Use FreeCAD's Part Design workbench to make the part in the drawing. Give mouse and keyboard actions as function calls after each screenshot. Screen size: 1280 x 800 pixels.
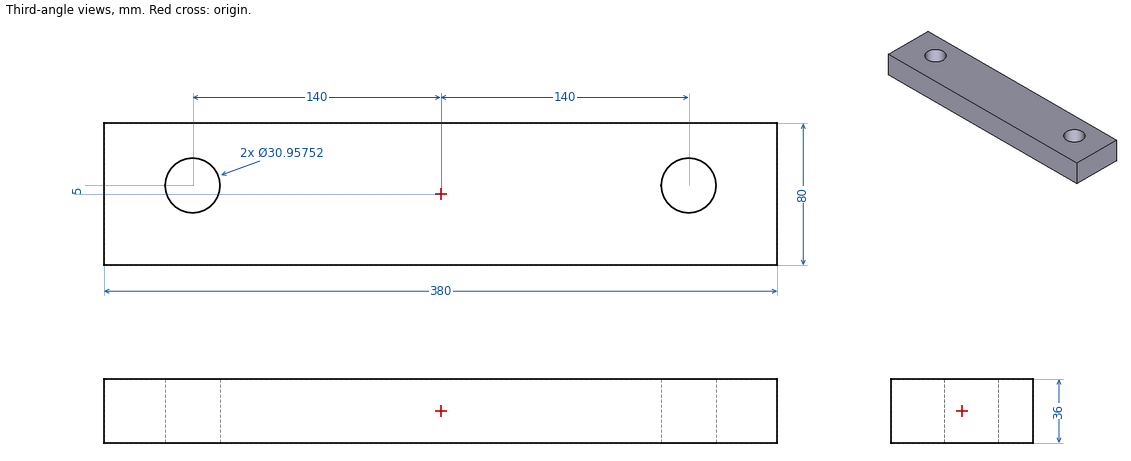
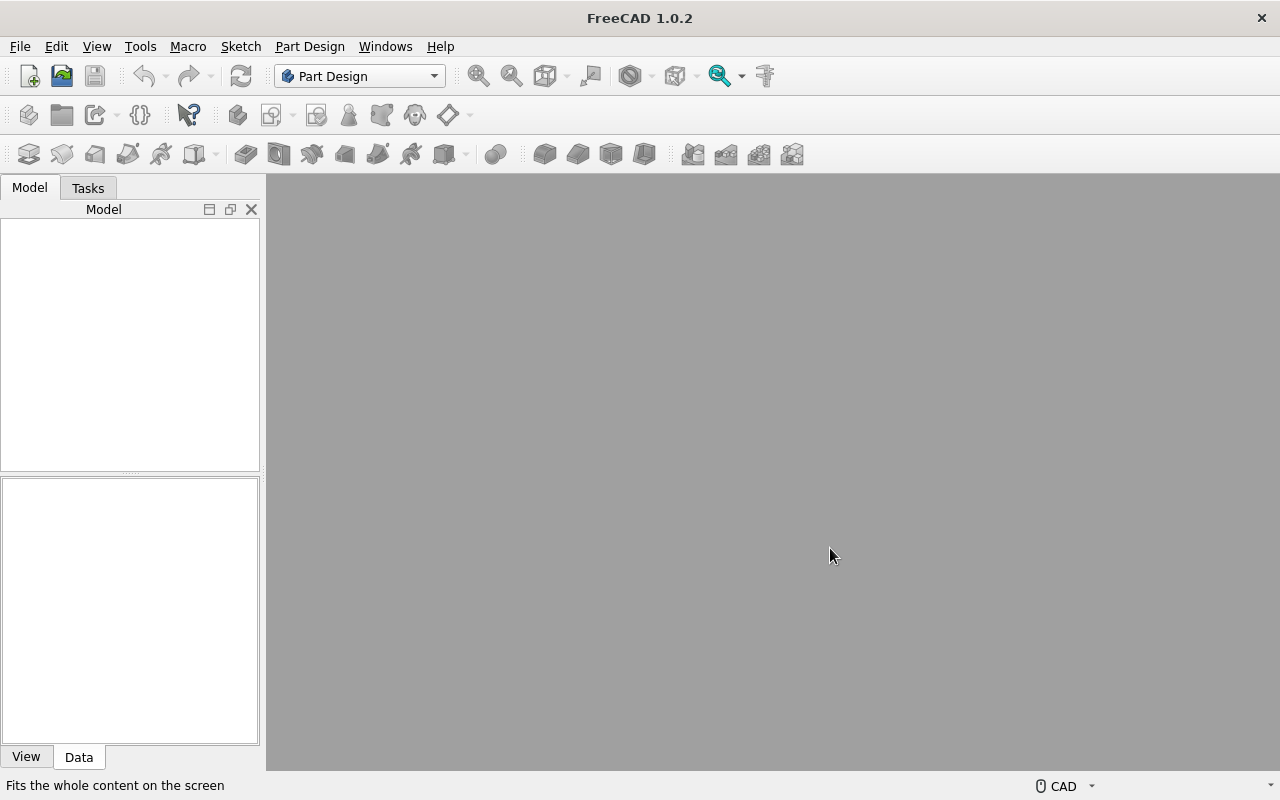
click(29, 76)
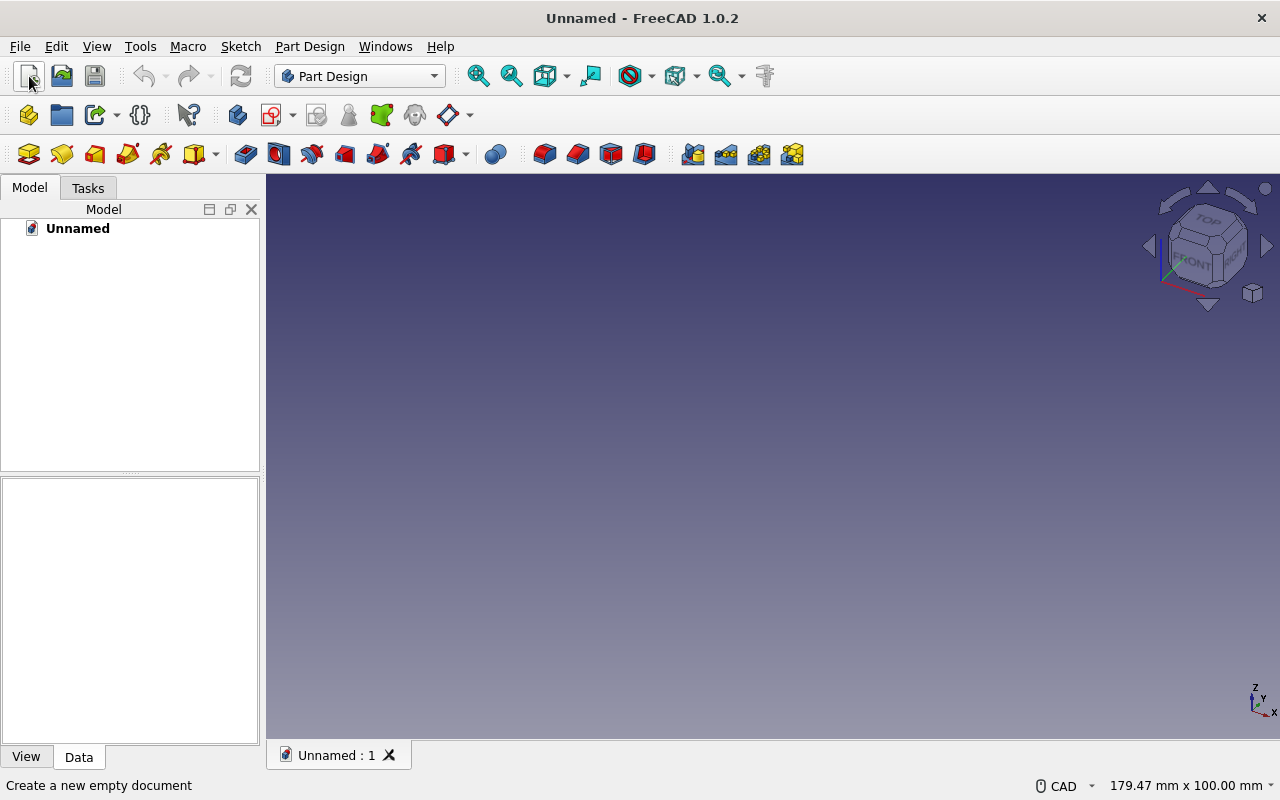
click(270, 116)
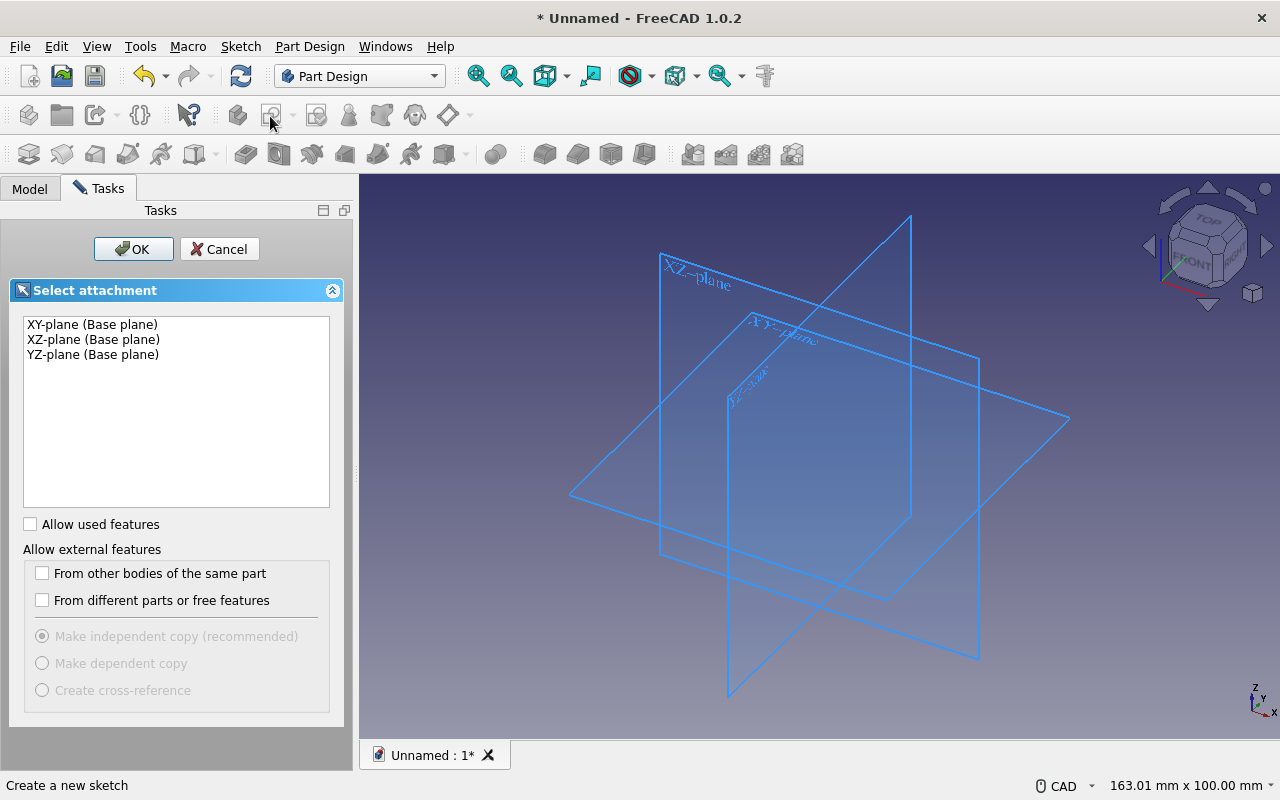
click(84, 324)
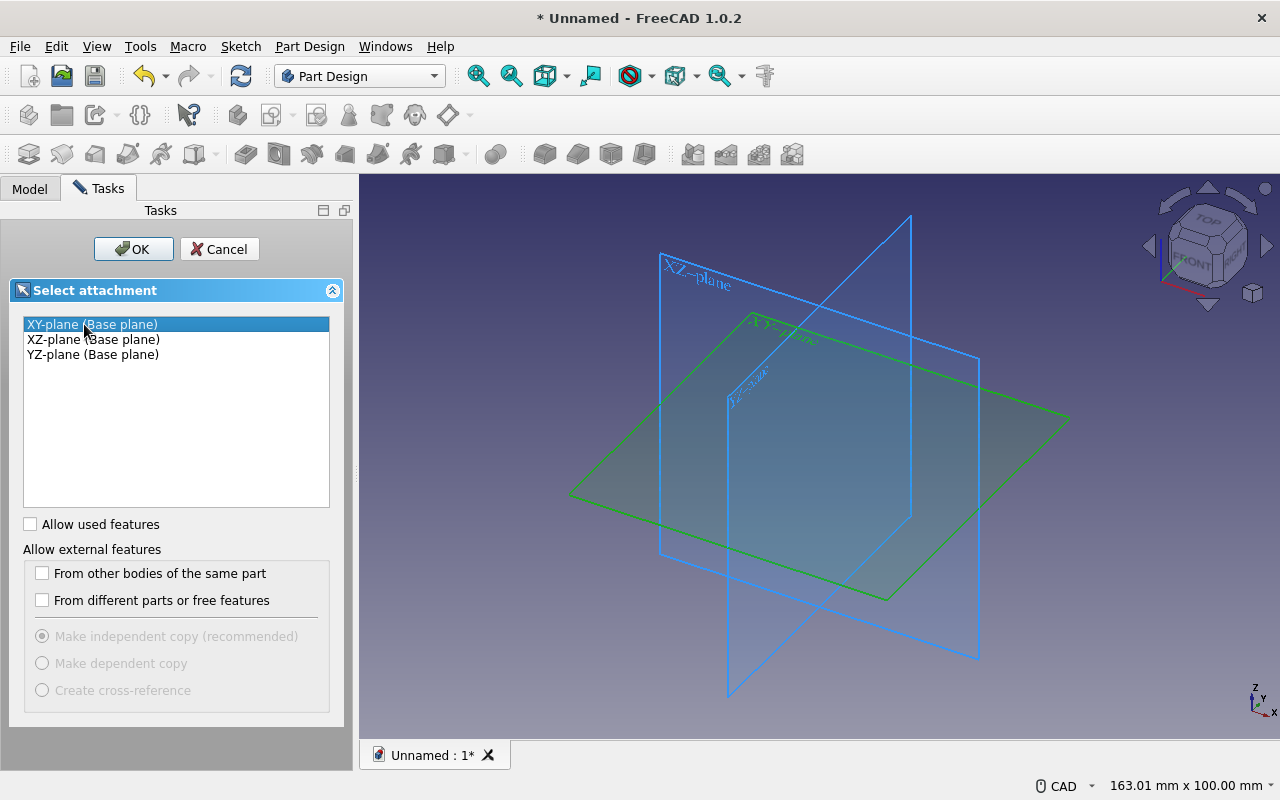
click(134, 249)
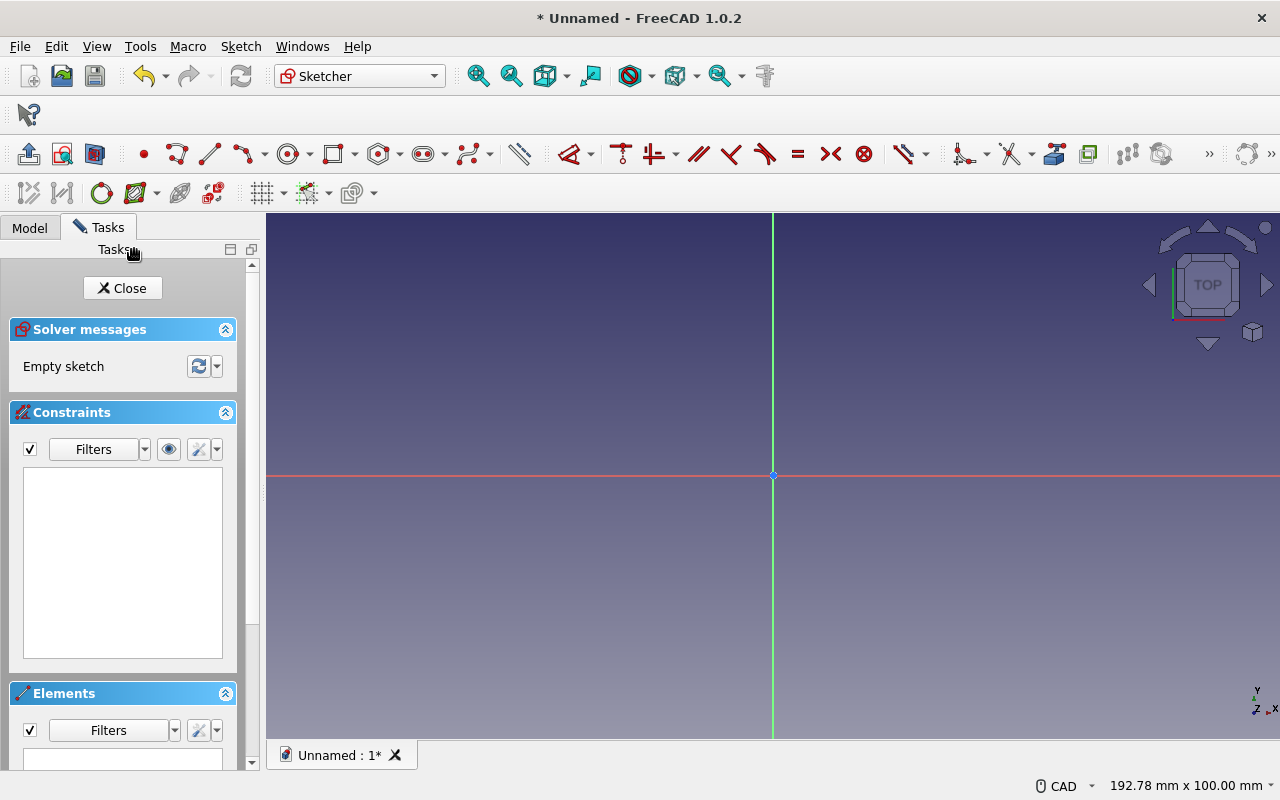
scroll(675, 476, down, 6)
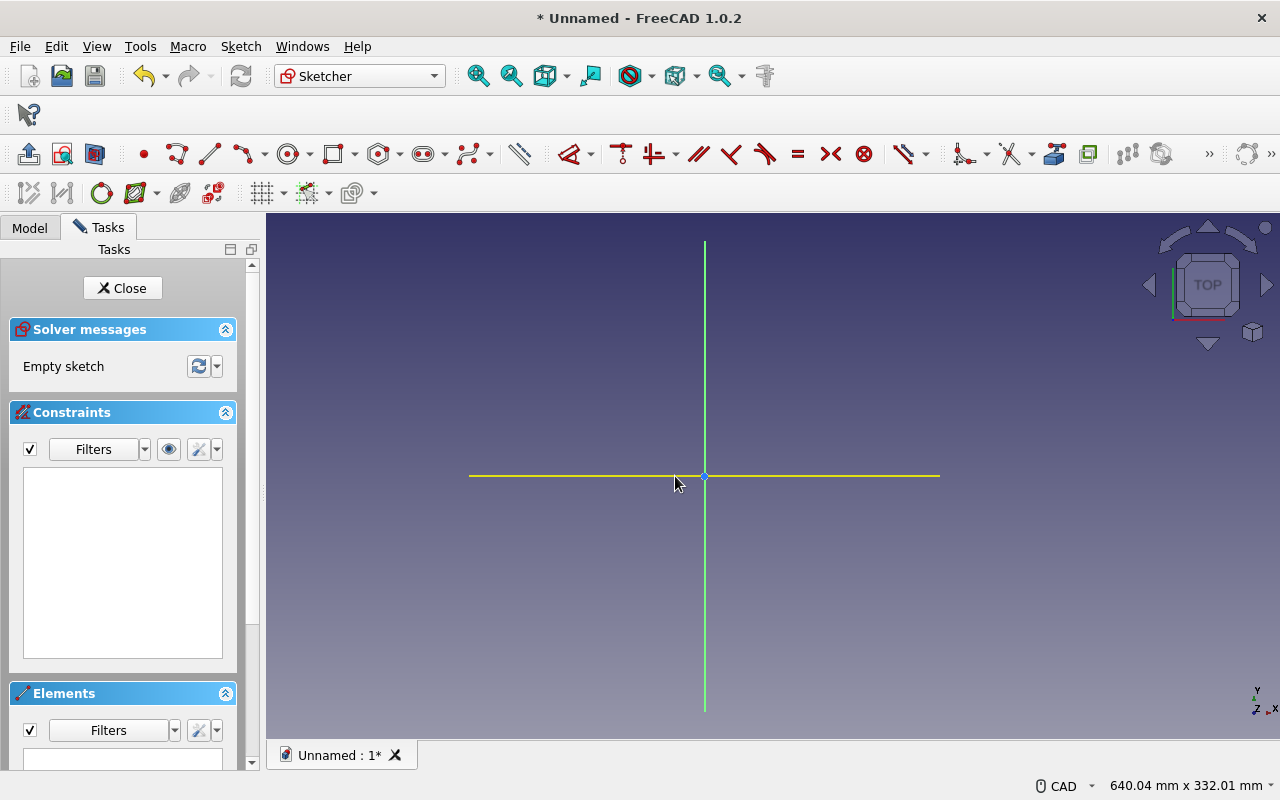
key(g)
key(v)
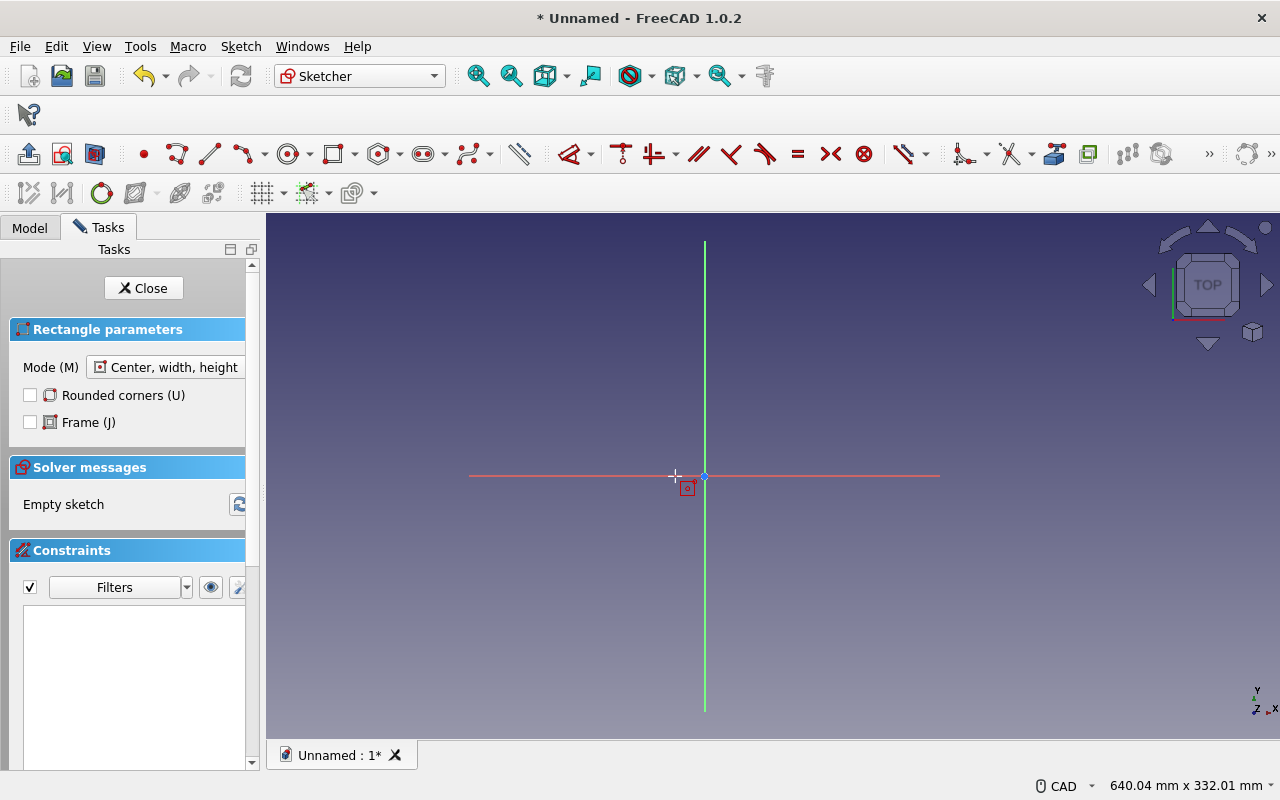
click(705, 476)
click(1006, 413)
key(Escape)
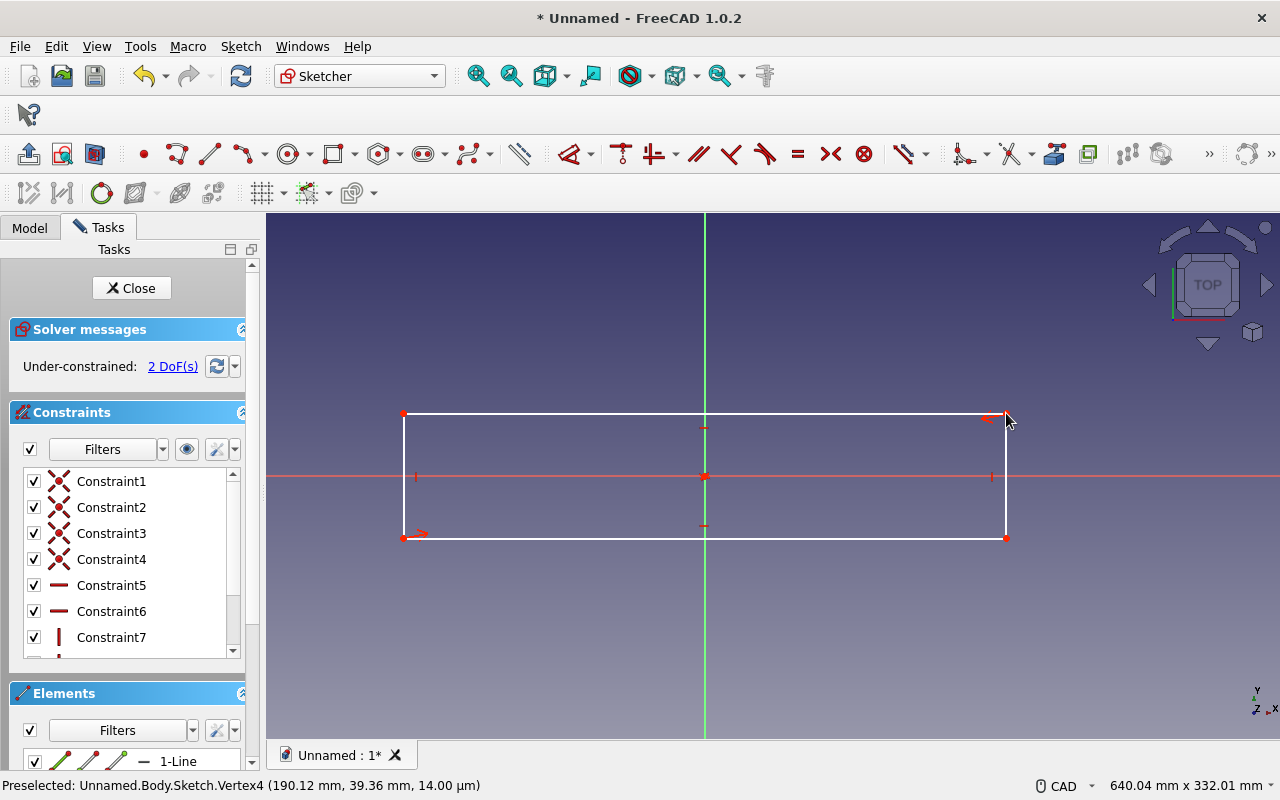
click(568, 154)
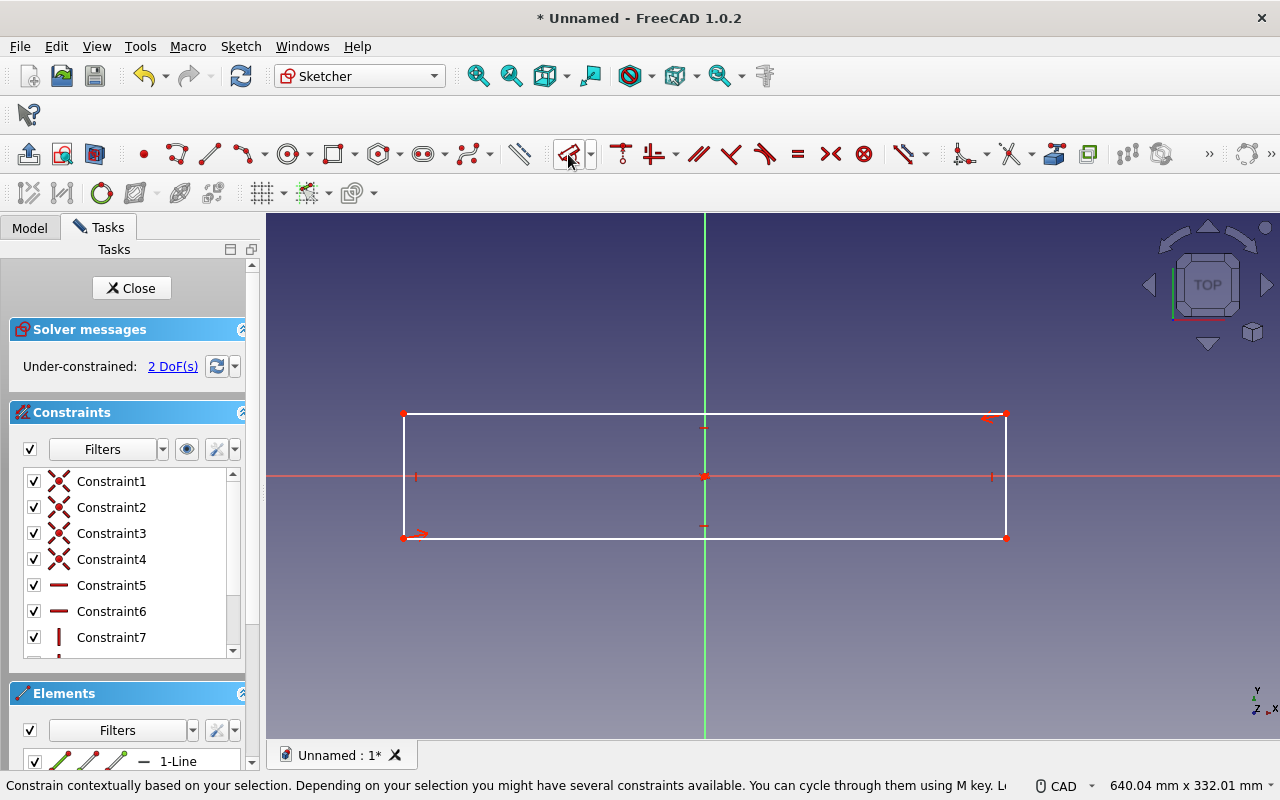
click(1006, 501)
click(1040, 448)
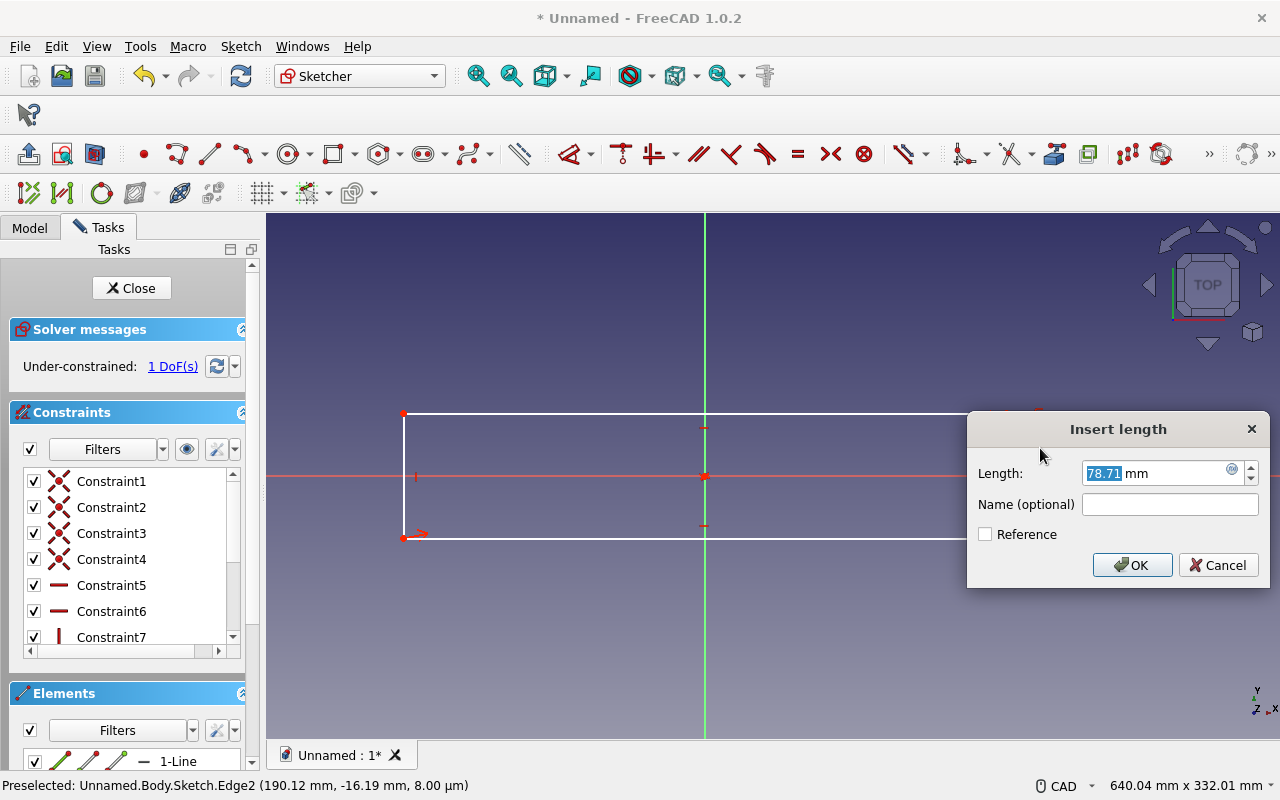
text(80)
key(Return)